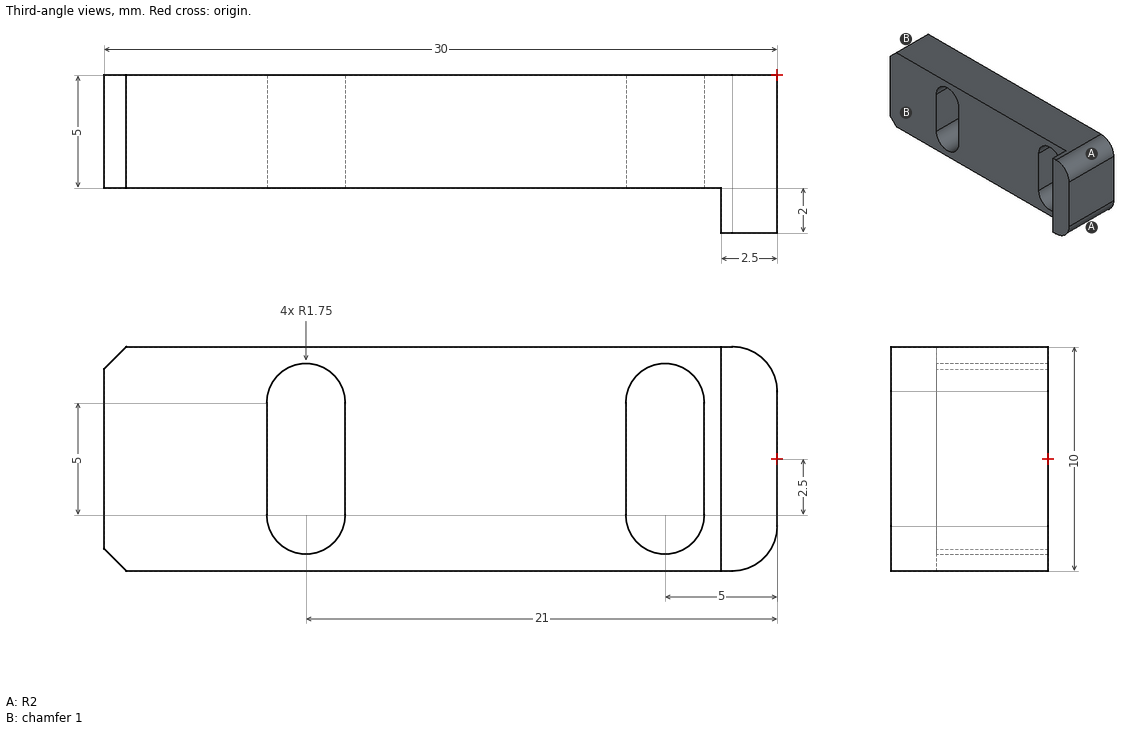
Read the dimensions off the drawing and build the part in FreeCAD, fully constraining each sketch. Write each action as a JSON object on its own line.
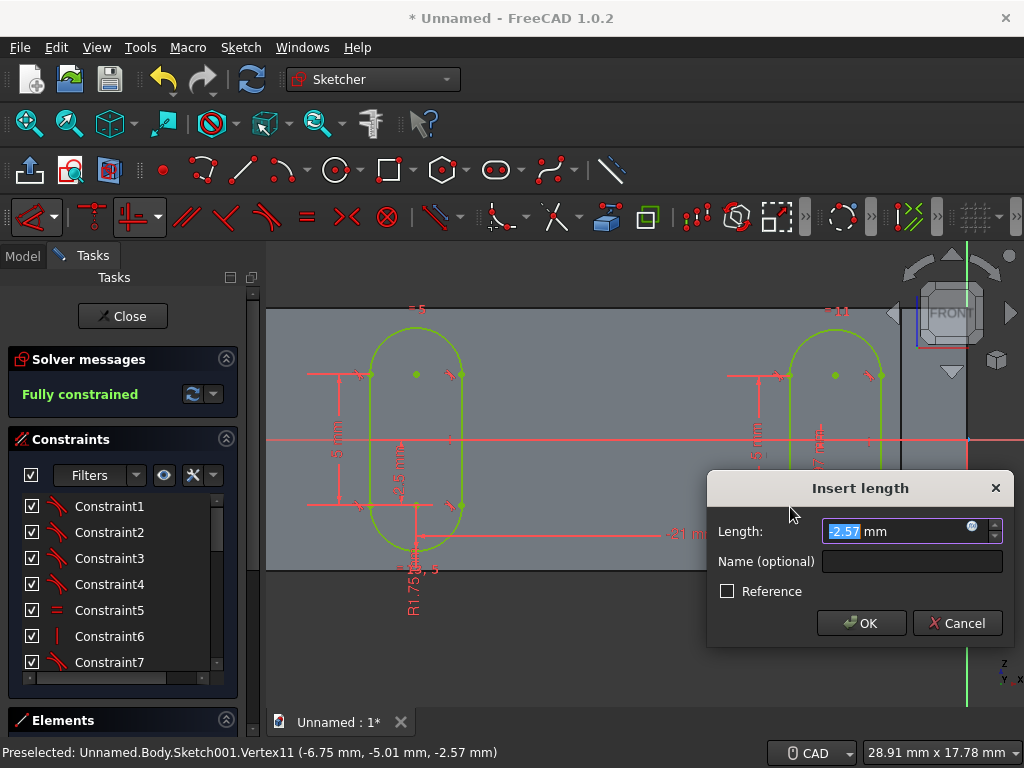
{"action": "type", "text": "-2.5"}
{"action": "key", "text": "Return"}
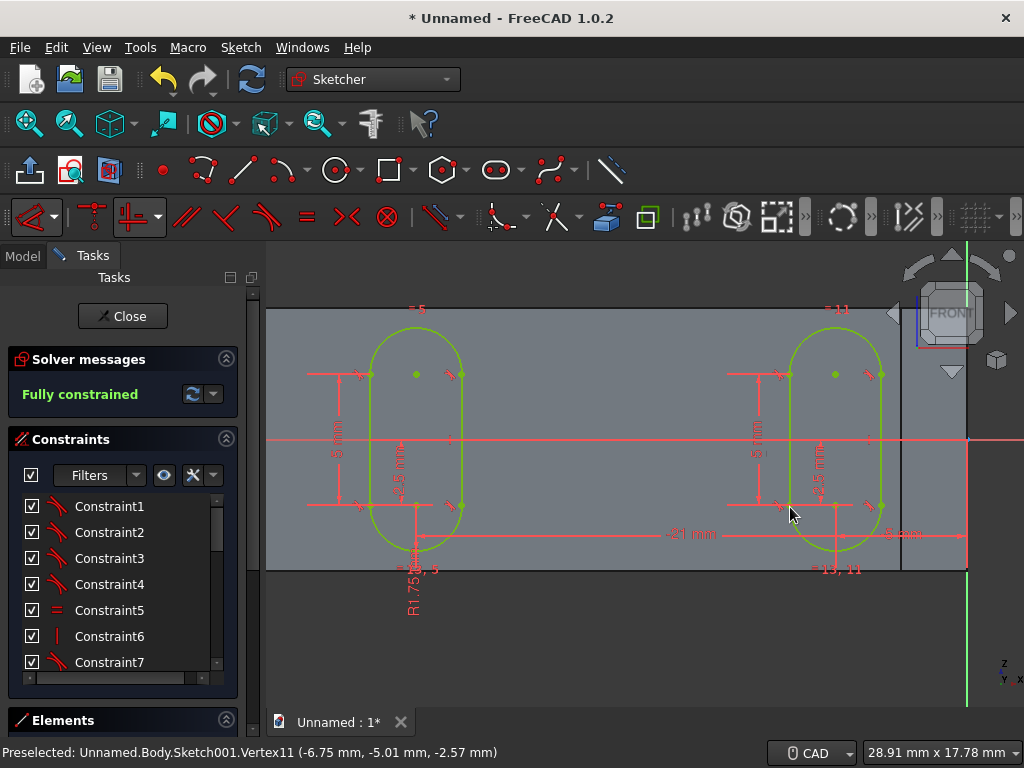
{"action": "left_click", "coordinate": [123, 316]}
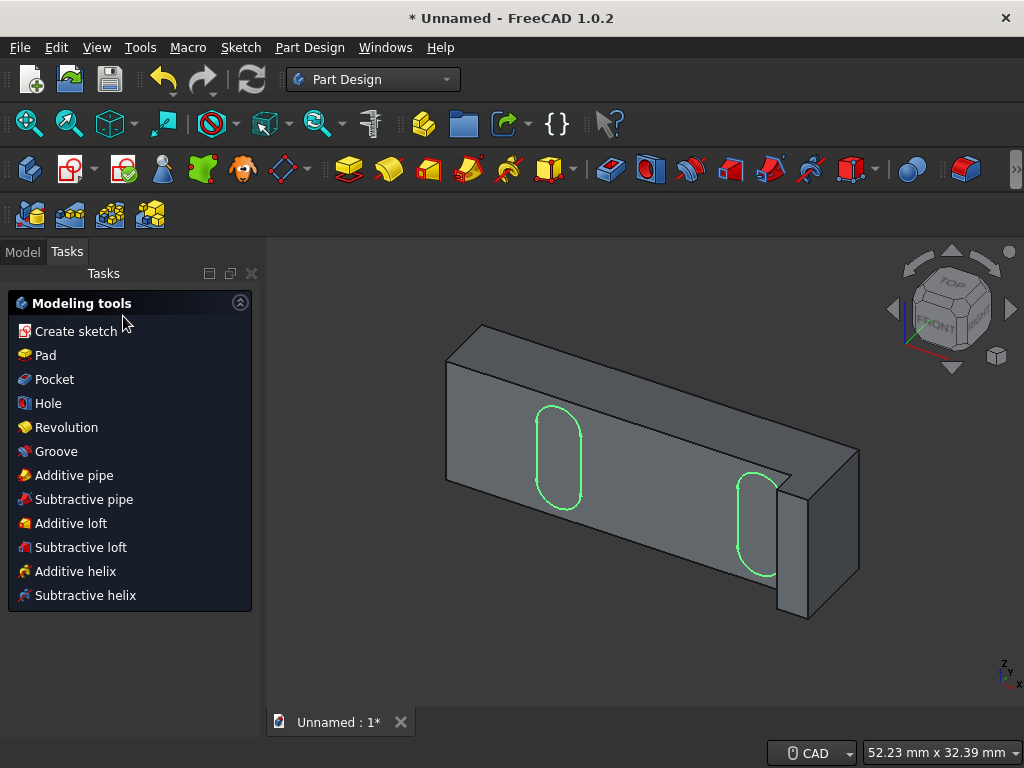
{"action": "left_click", "coordinate": [612, 170]}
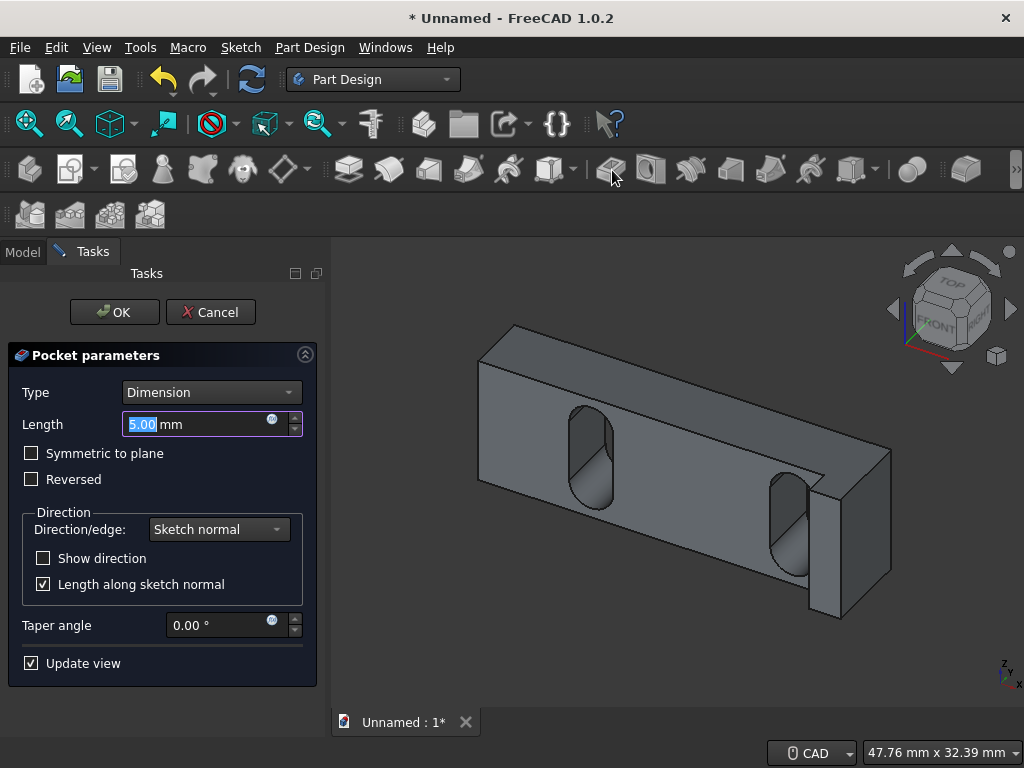
{"action": "left_click", "coordinate": [212, 392]}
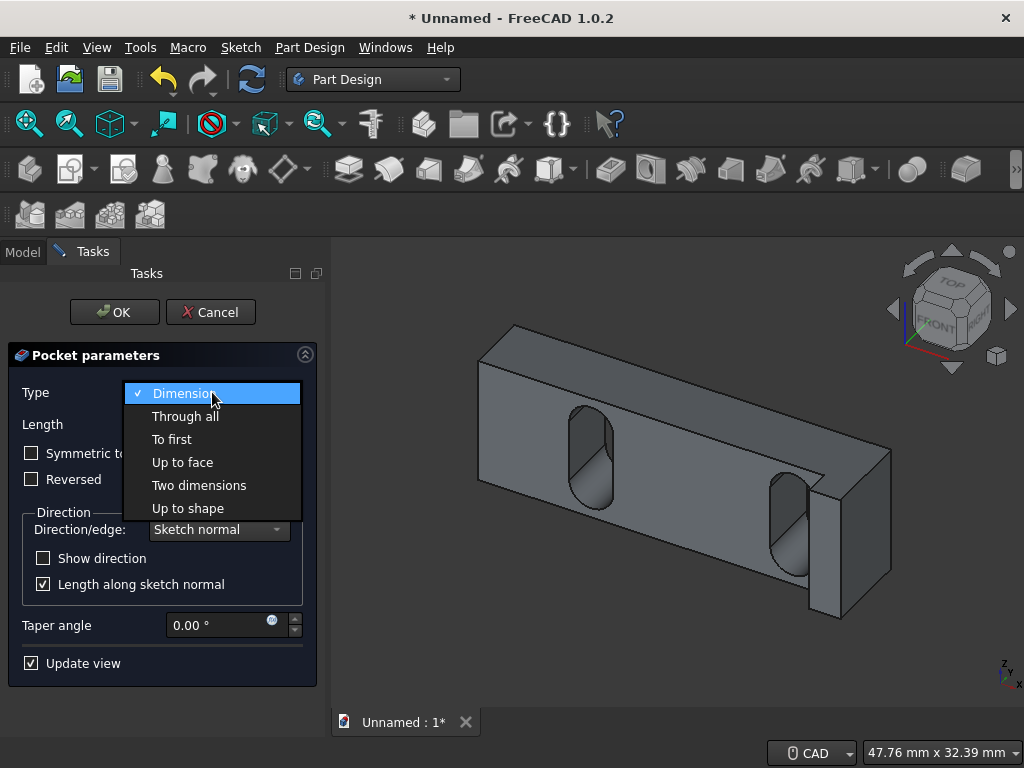
{"action": "left_click", "coordinate": [212, 416]}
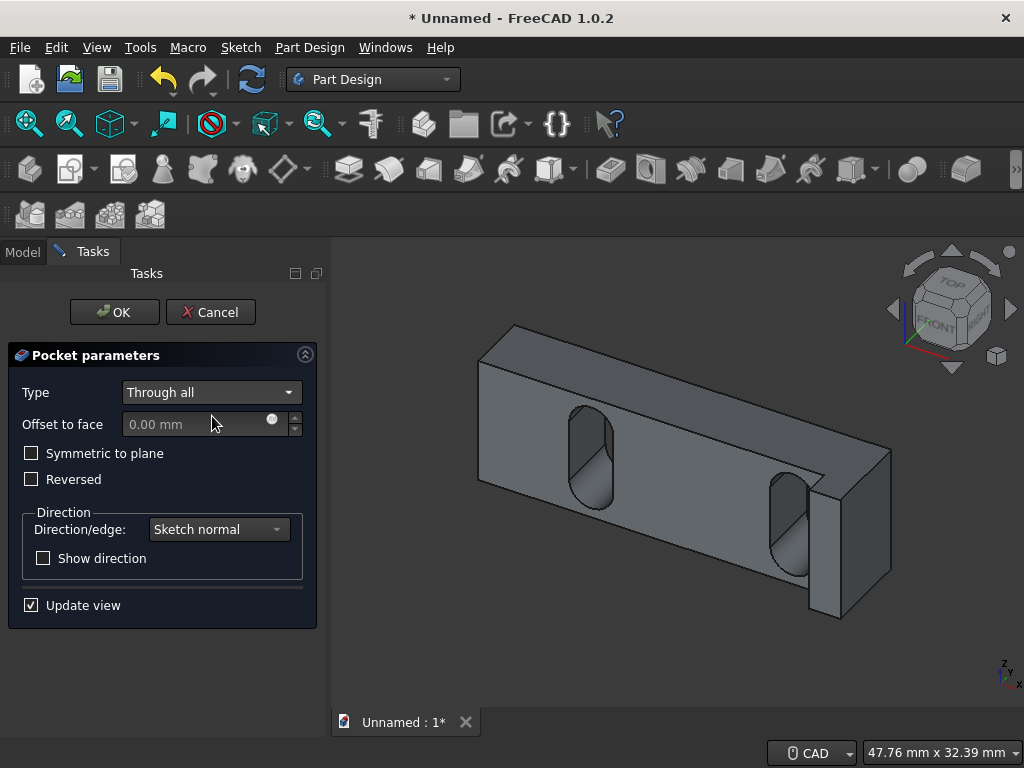
{"action": "left_click", "coordinate": [115, 312]}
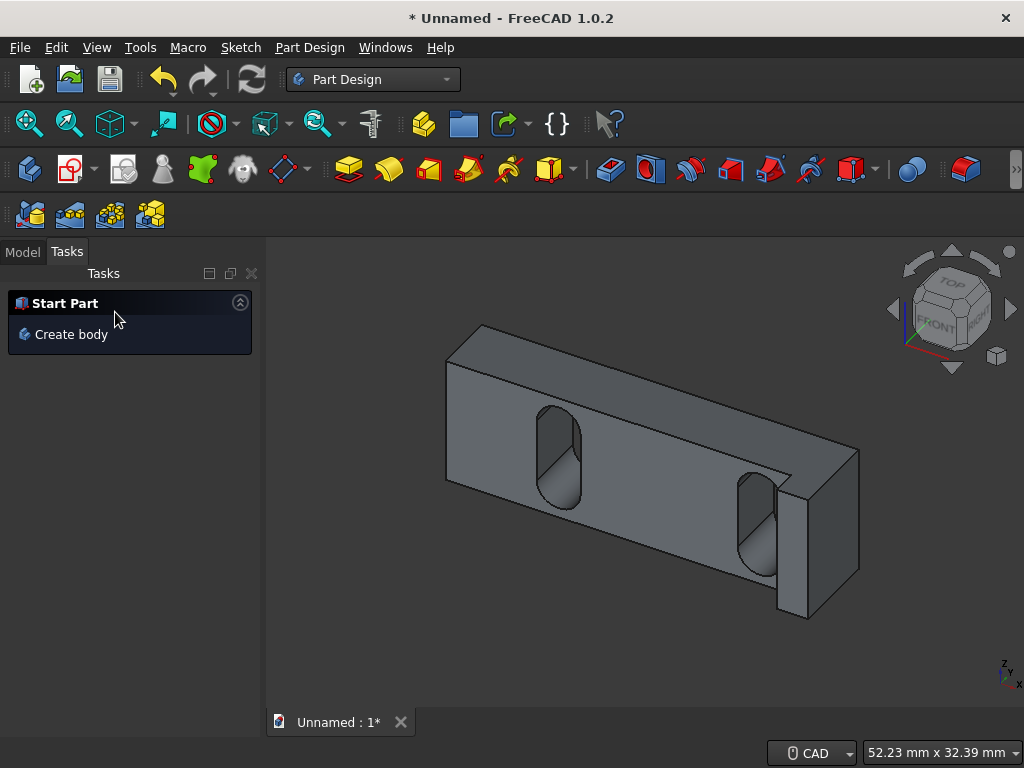
{"action": "left_click", "coordinate": [834, 474]}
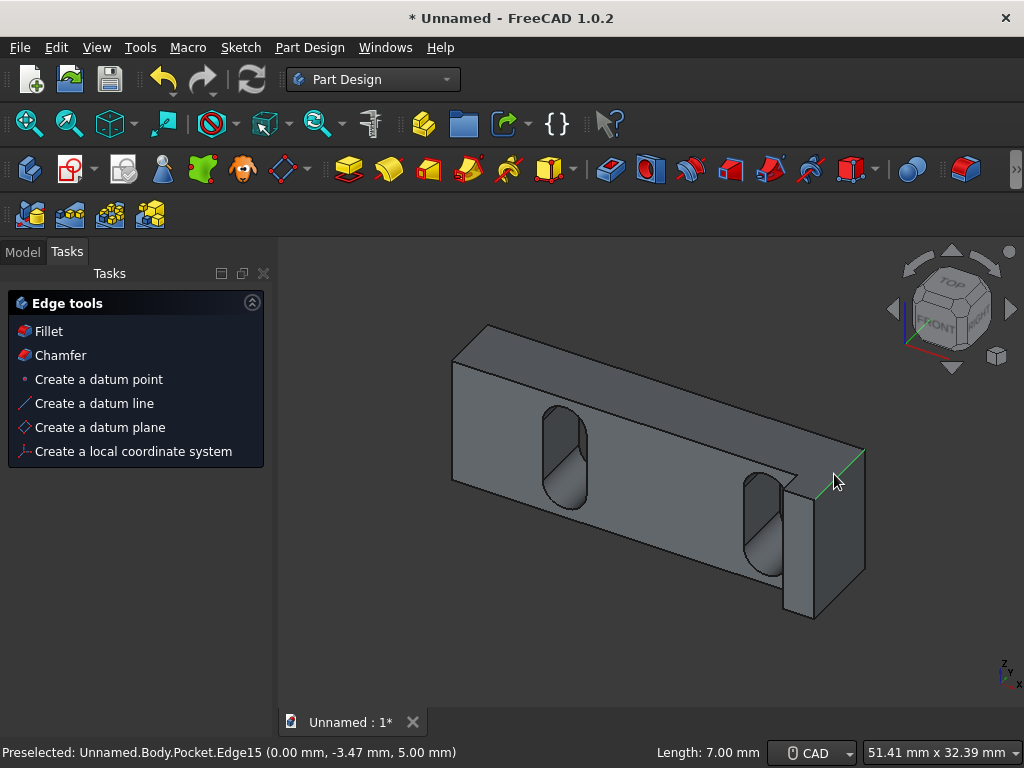
{"action": "key", "text": "0"}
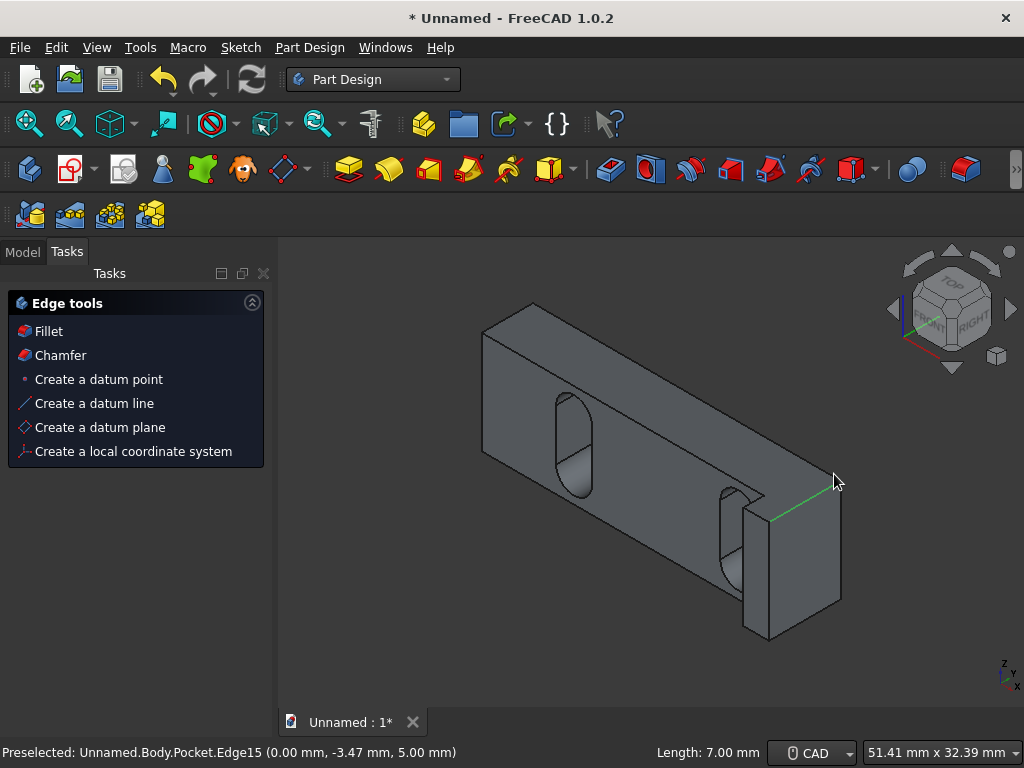
{"action": "key", "text": "2"}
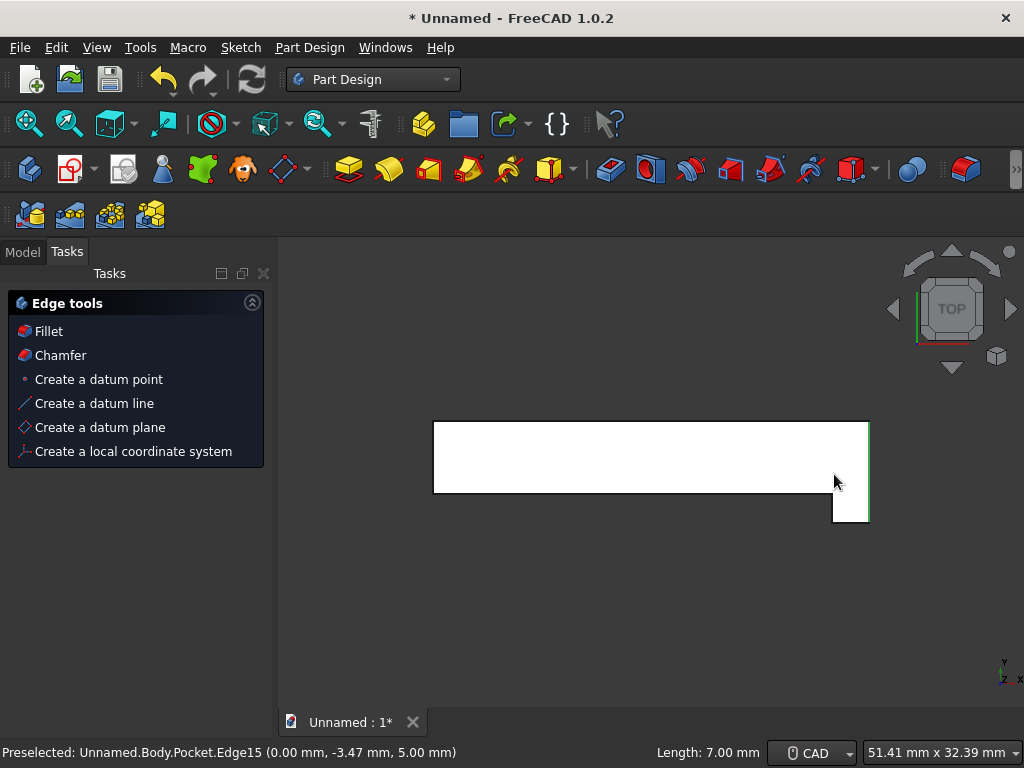
{"action": "key", "text": "1"}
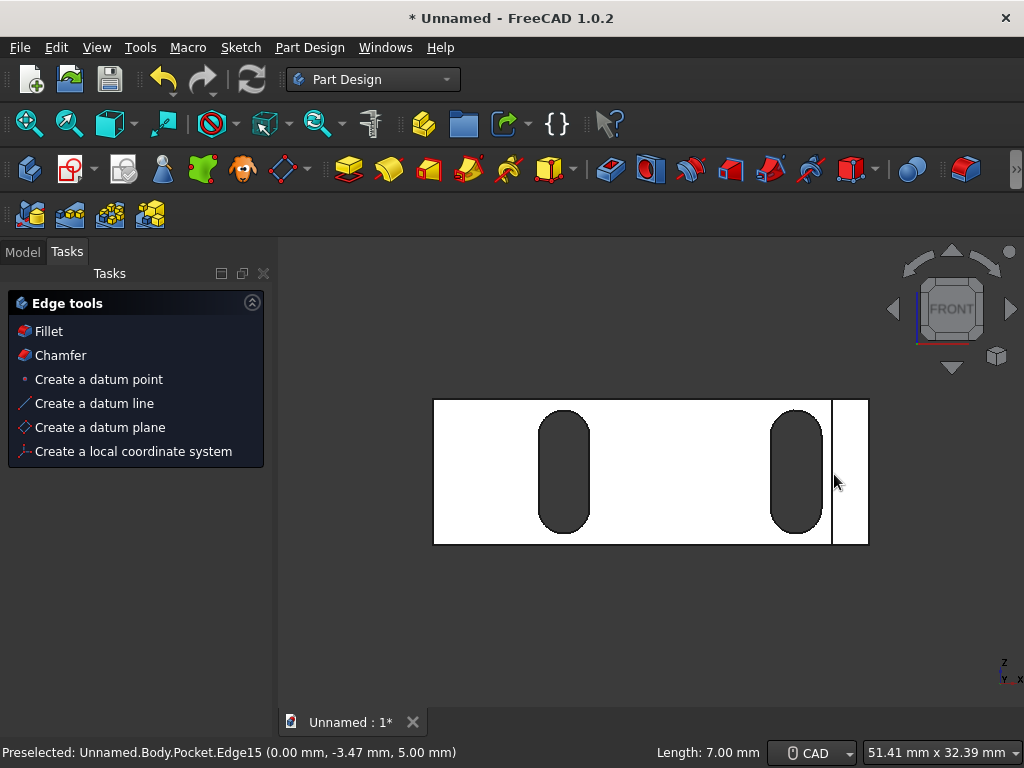
{"action": "key", "text": "3"}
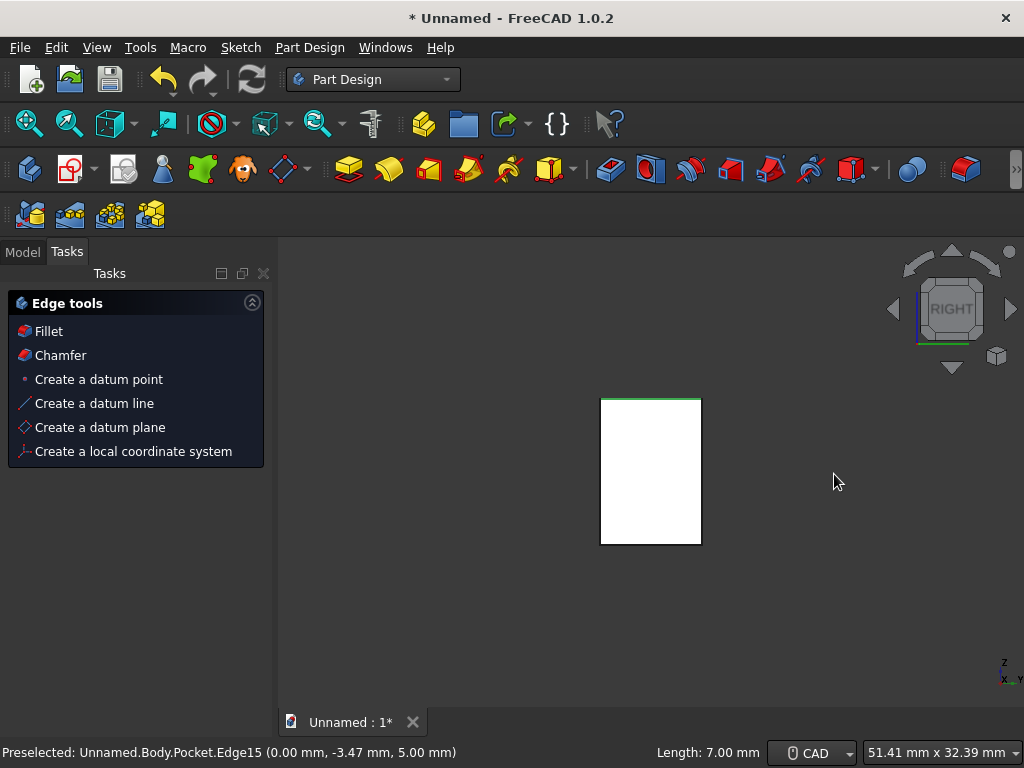
{"action": "left_click", "coordinate": [30, 124]}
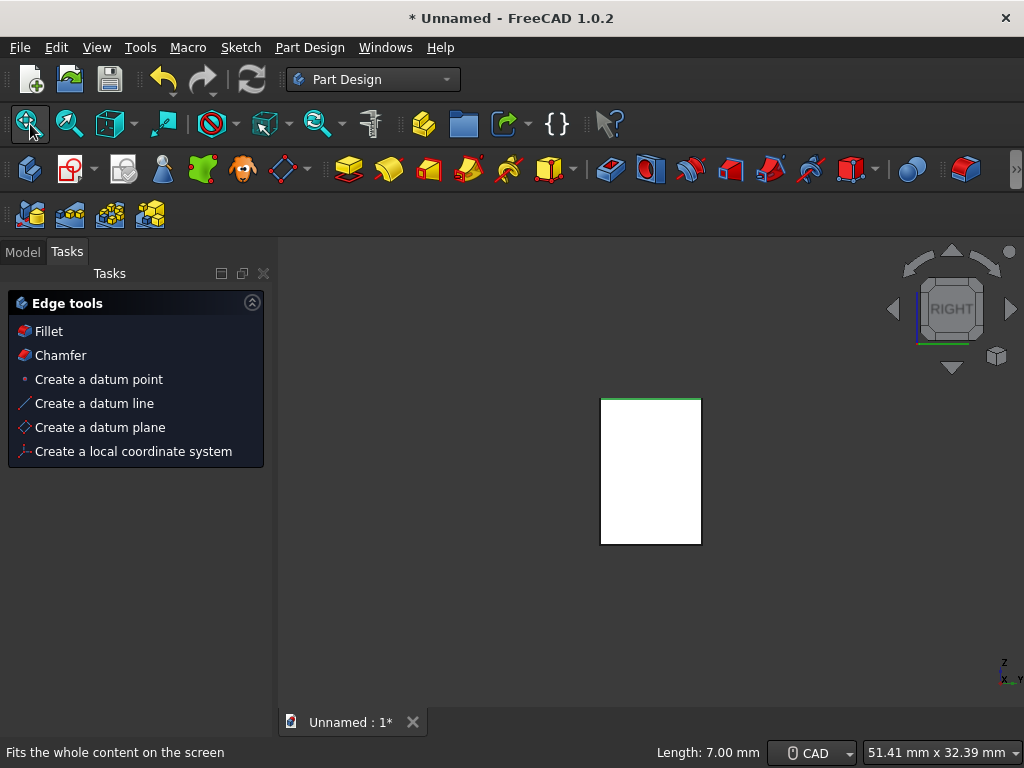
{"action": "left_click", "coordinate": [651, 544], "text": "ctrl"}